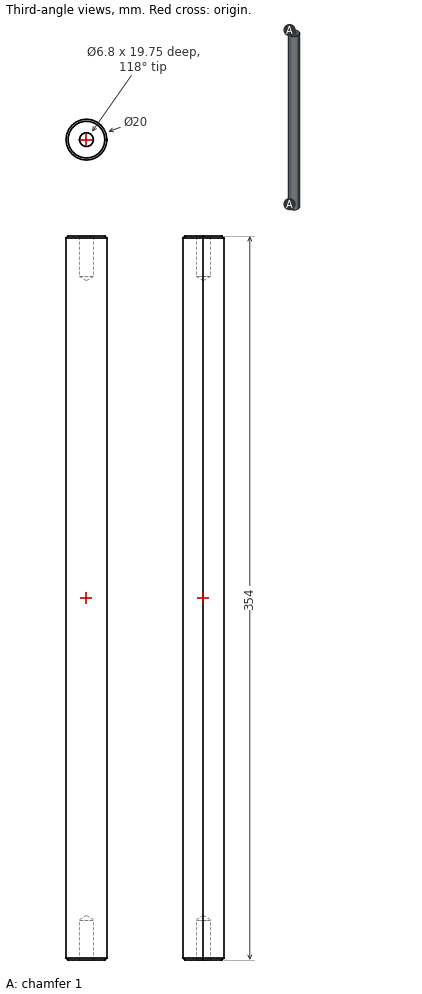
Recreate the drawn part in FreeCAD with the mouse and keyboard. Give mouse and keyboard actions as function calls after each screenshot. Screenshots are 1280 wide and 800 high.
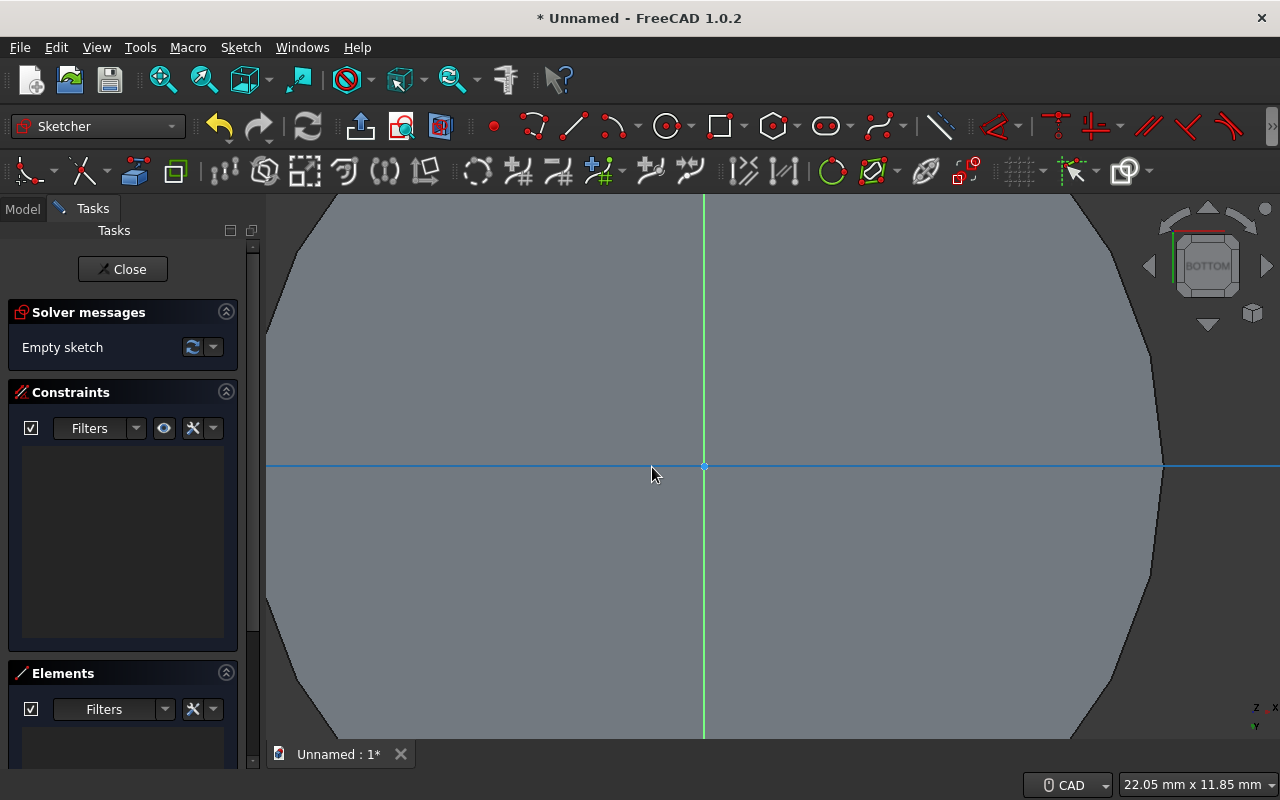
key(g)
key(c)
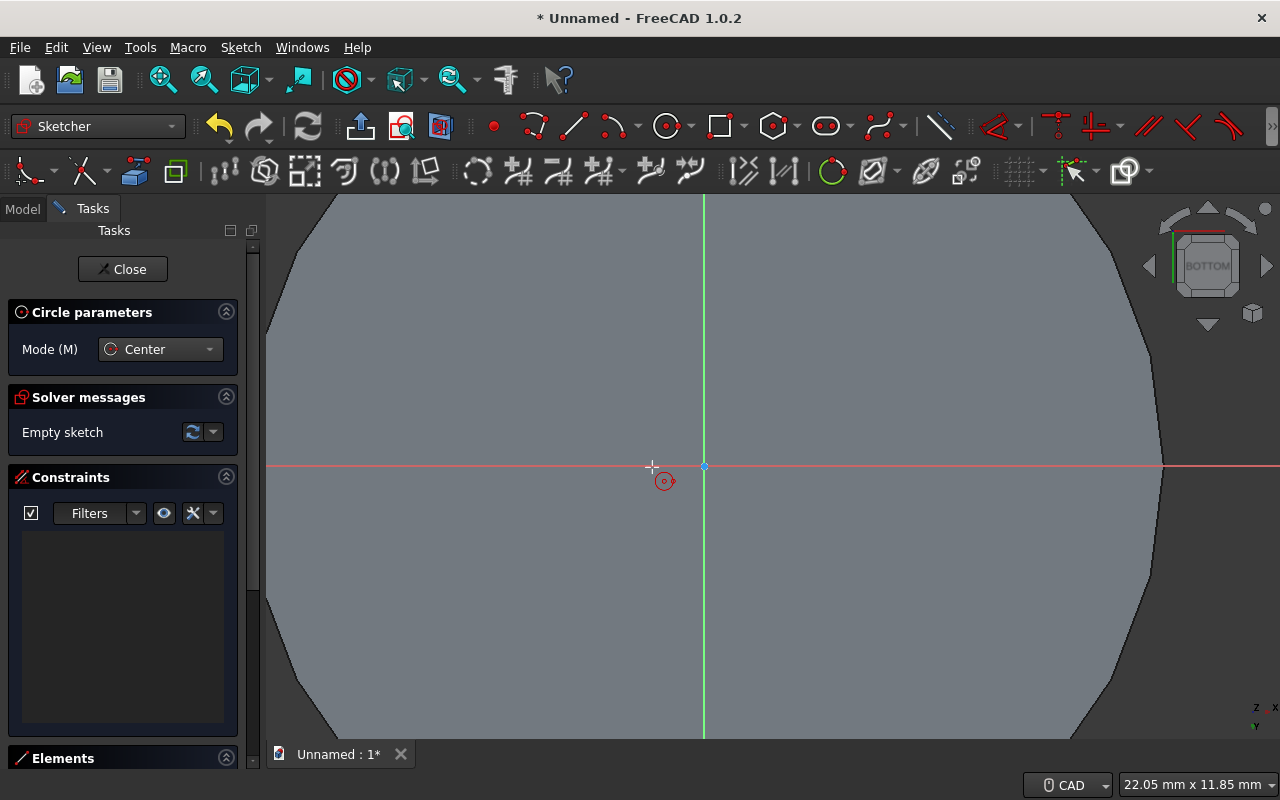
click(704, 466)
move(815, 355)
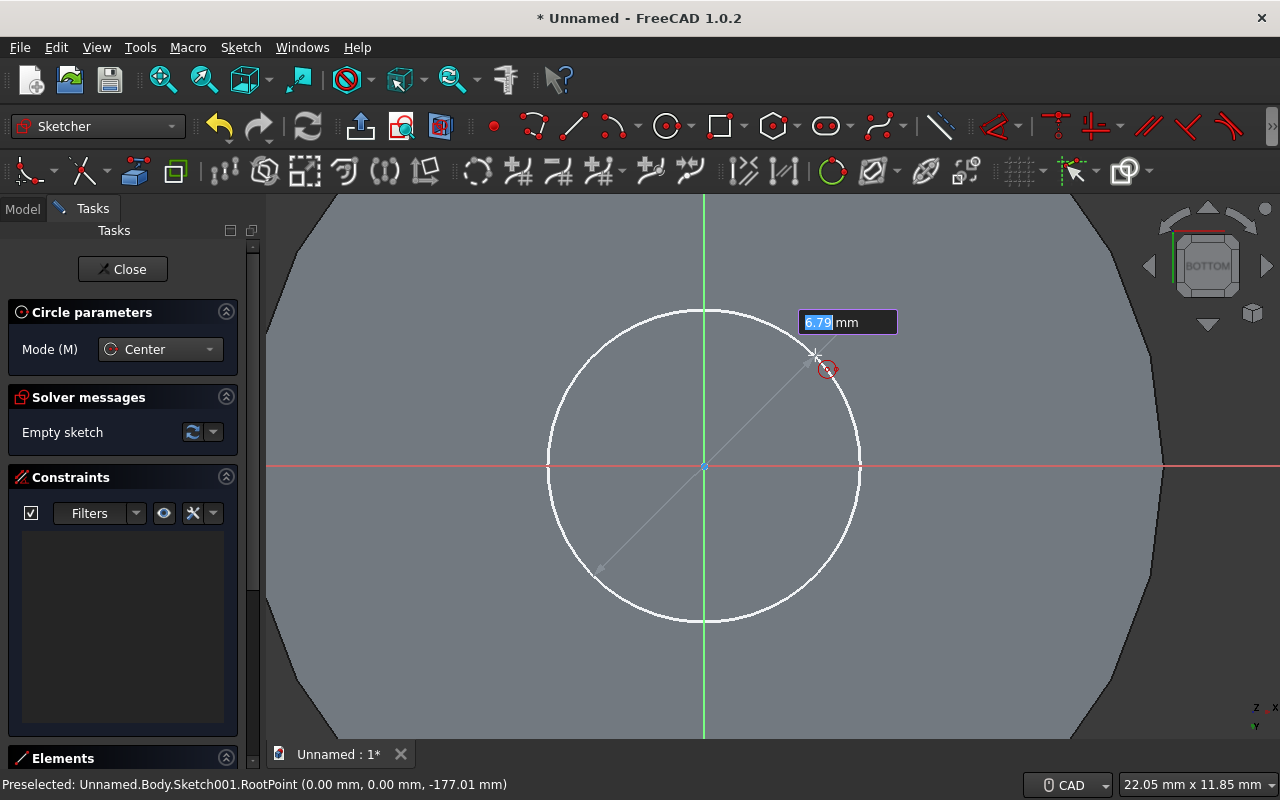
text(6.8)
key(Return)
key(Escape)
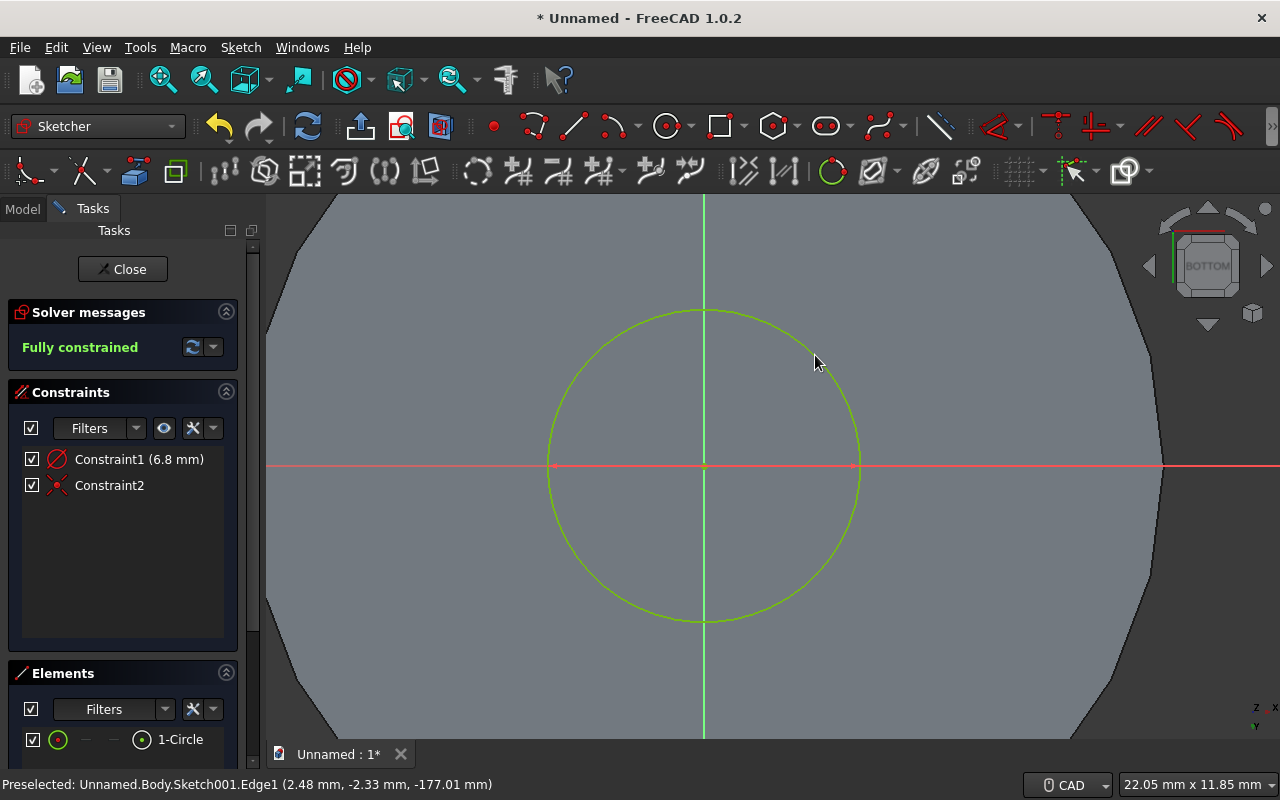
click(123, 269)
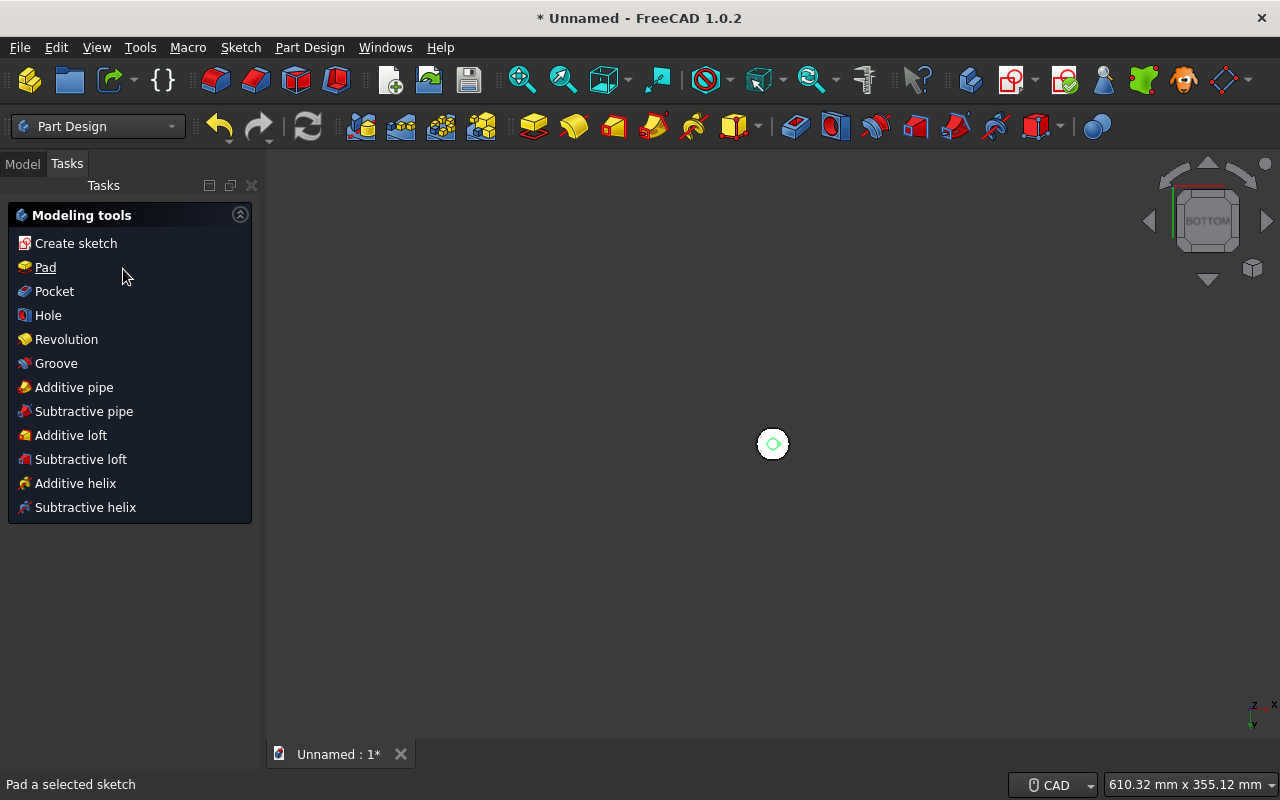
click(836, 126)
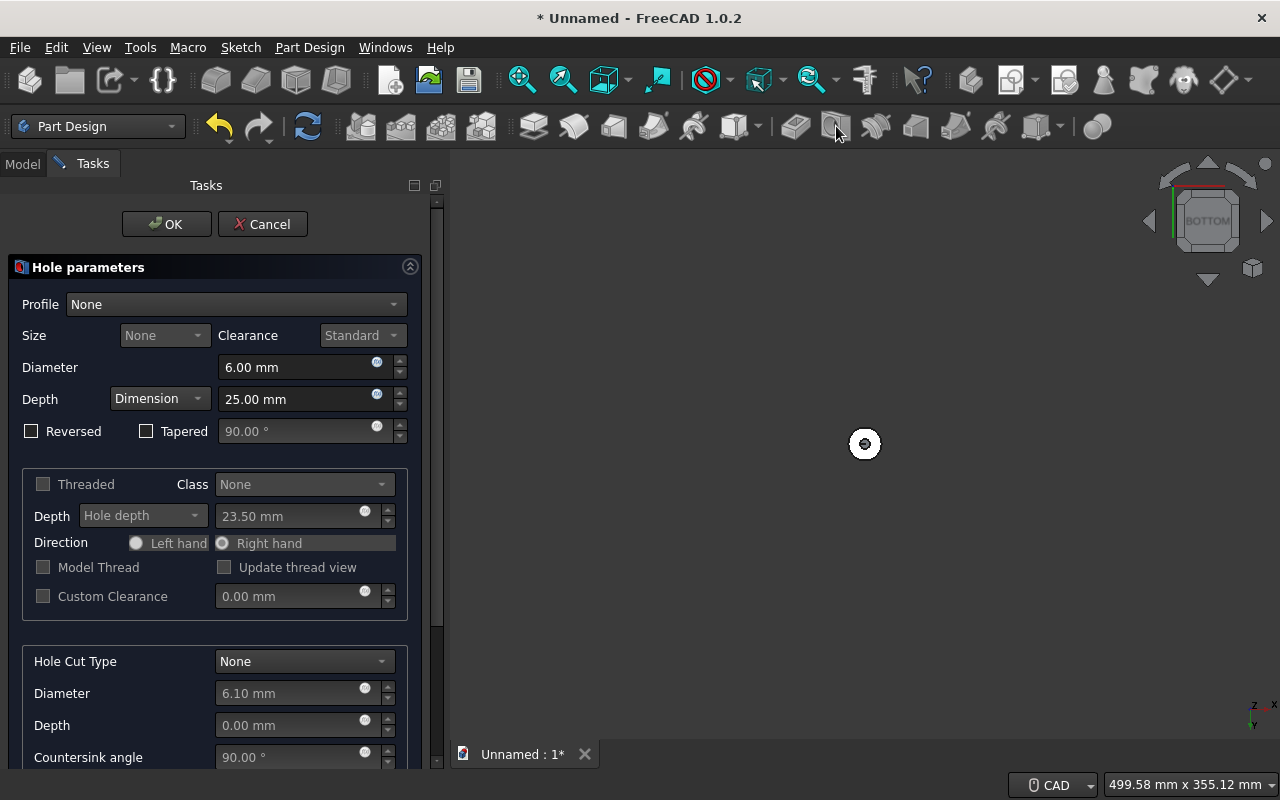
triple_click(305, 367)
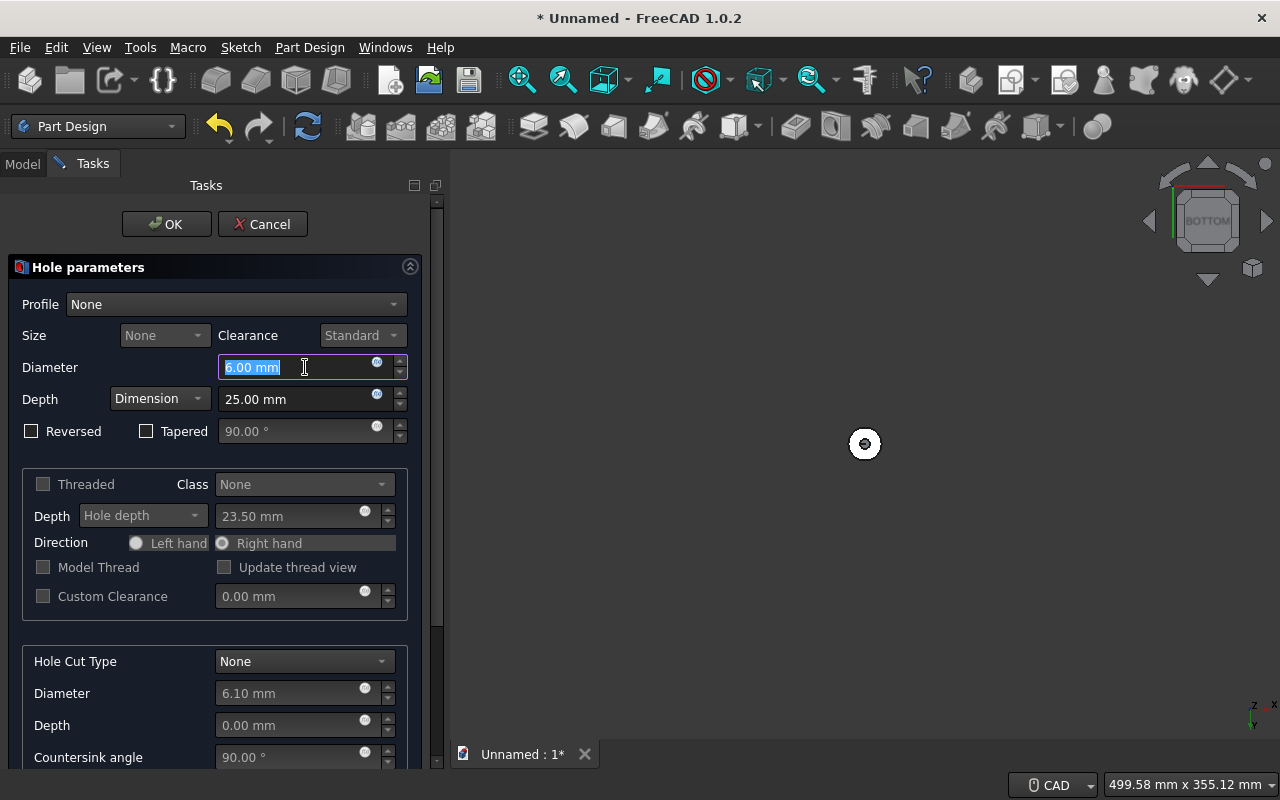
text(6.8)
key(Tab)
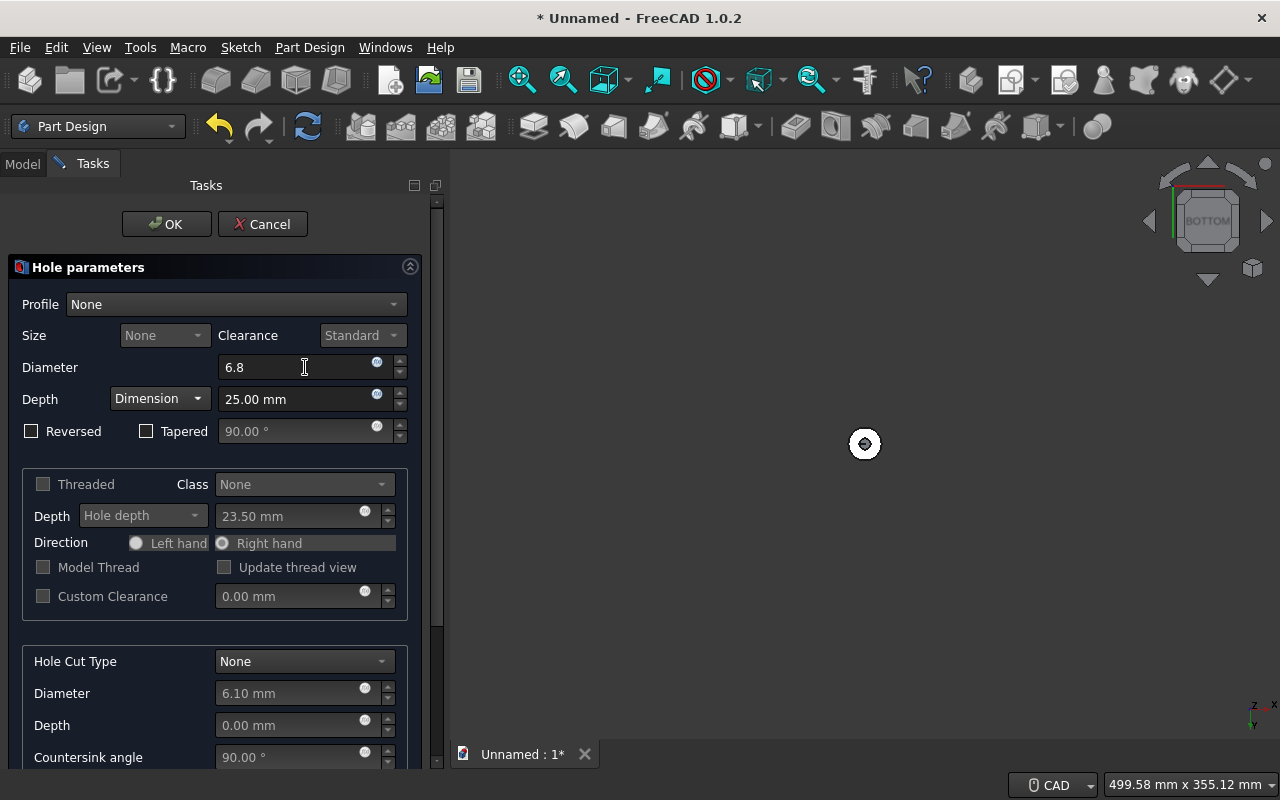
triple_click(305, 399)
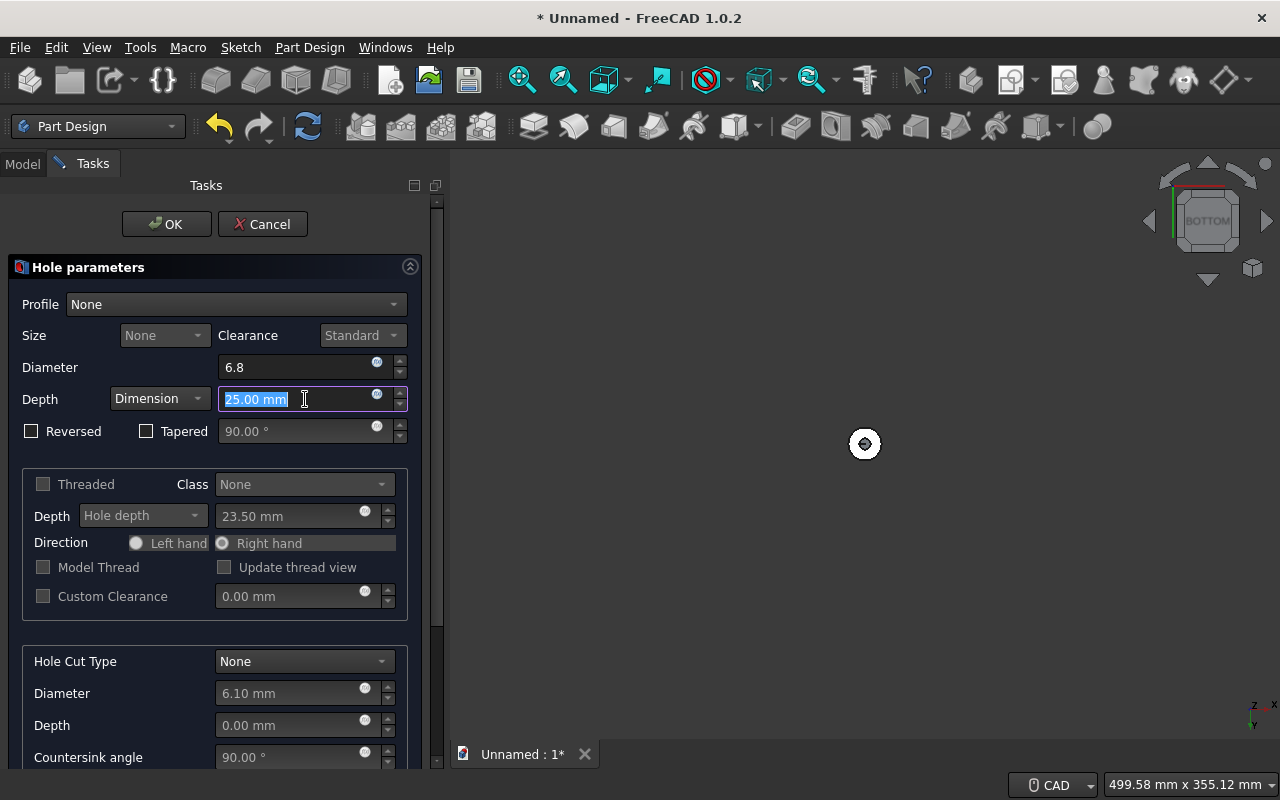
text(19.75)
key(Tab)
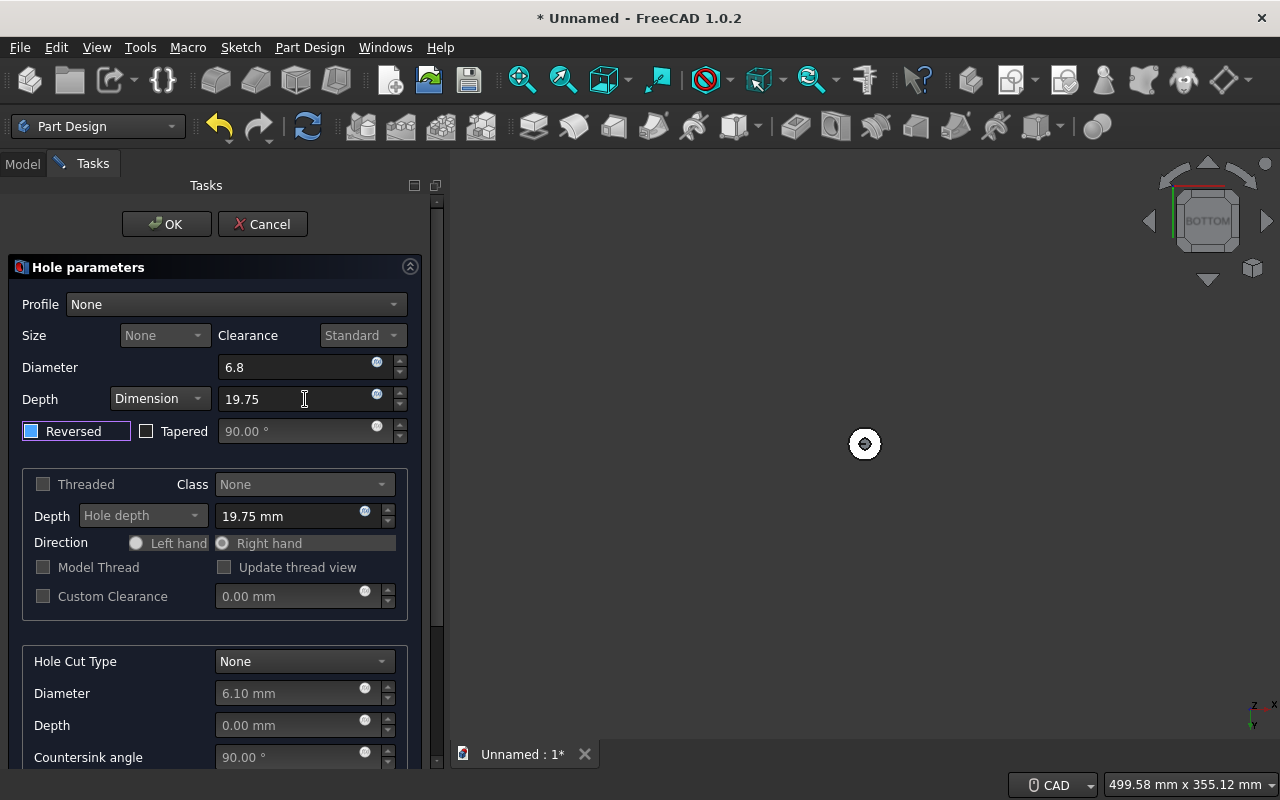
click(167, 224)